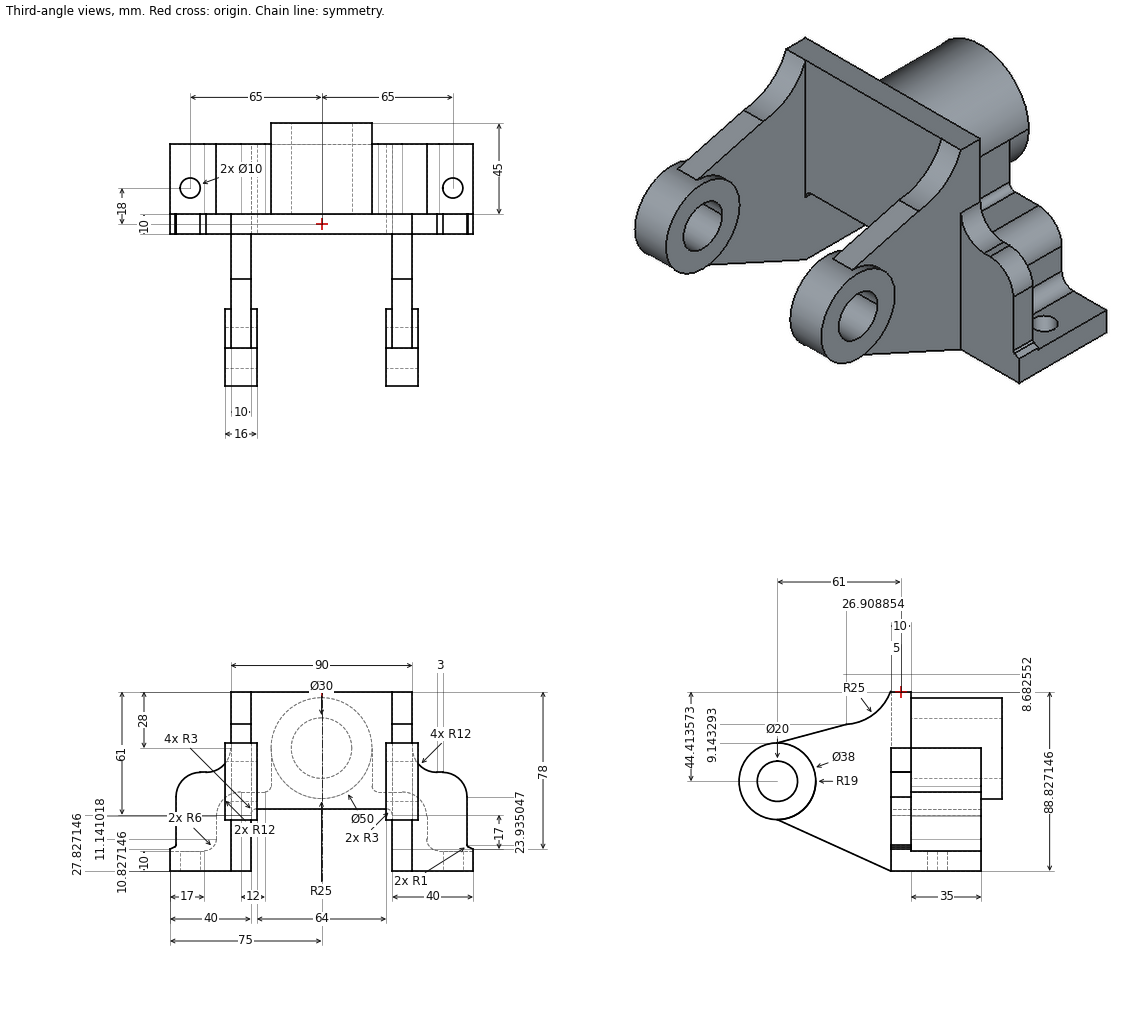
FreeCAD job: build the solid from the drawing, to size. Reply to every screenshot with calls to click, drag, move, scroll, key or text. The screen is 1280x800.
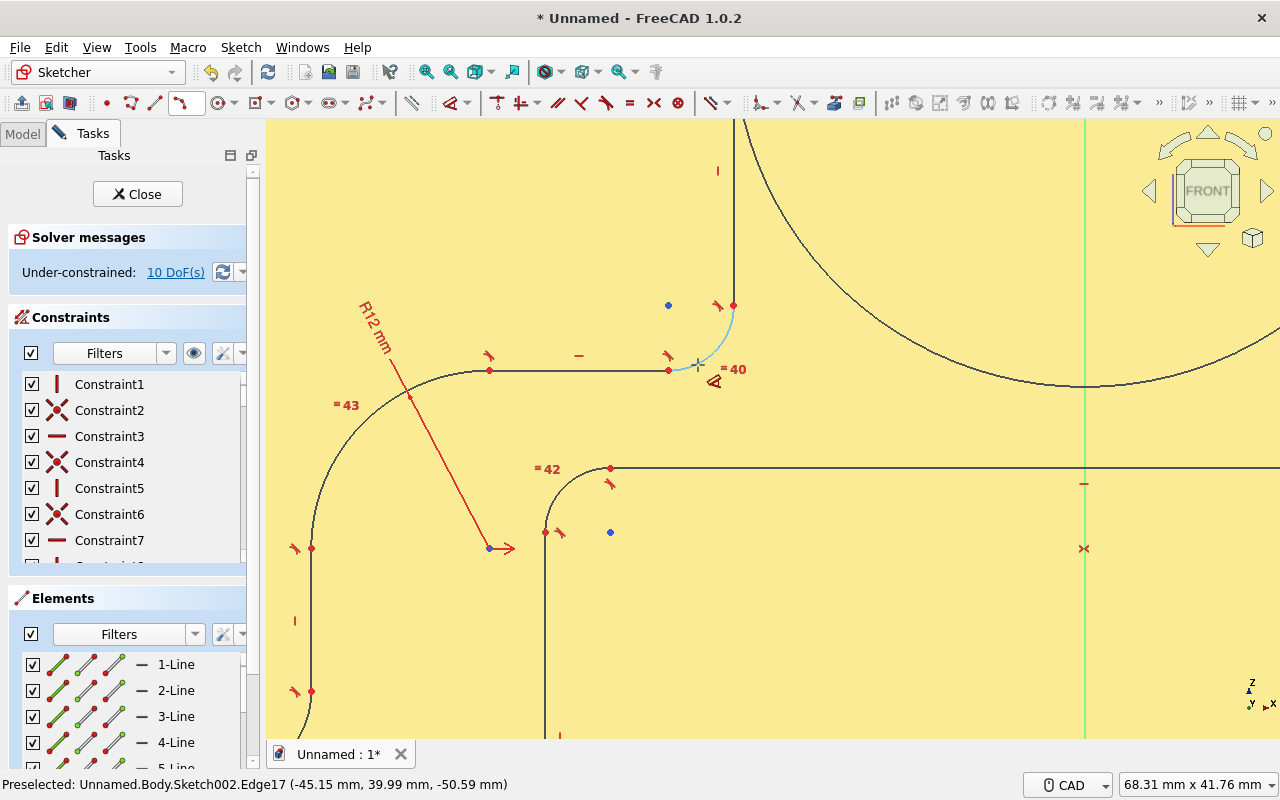
click(698, 364)
click(712, 393)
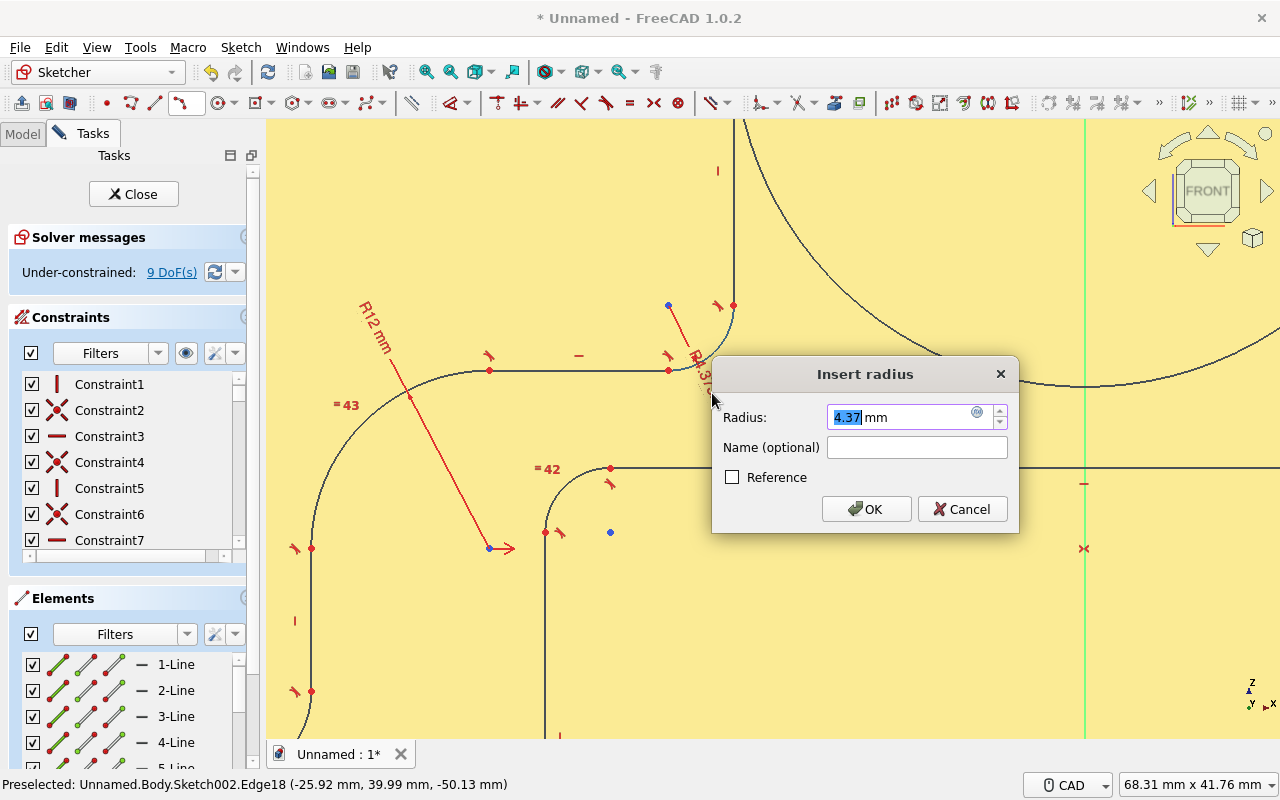
text(3)
key(Return)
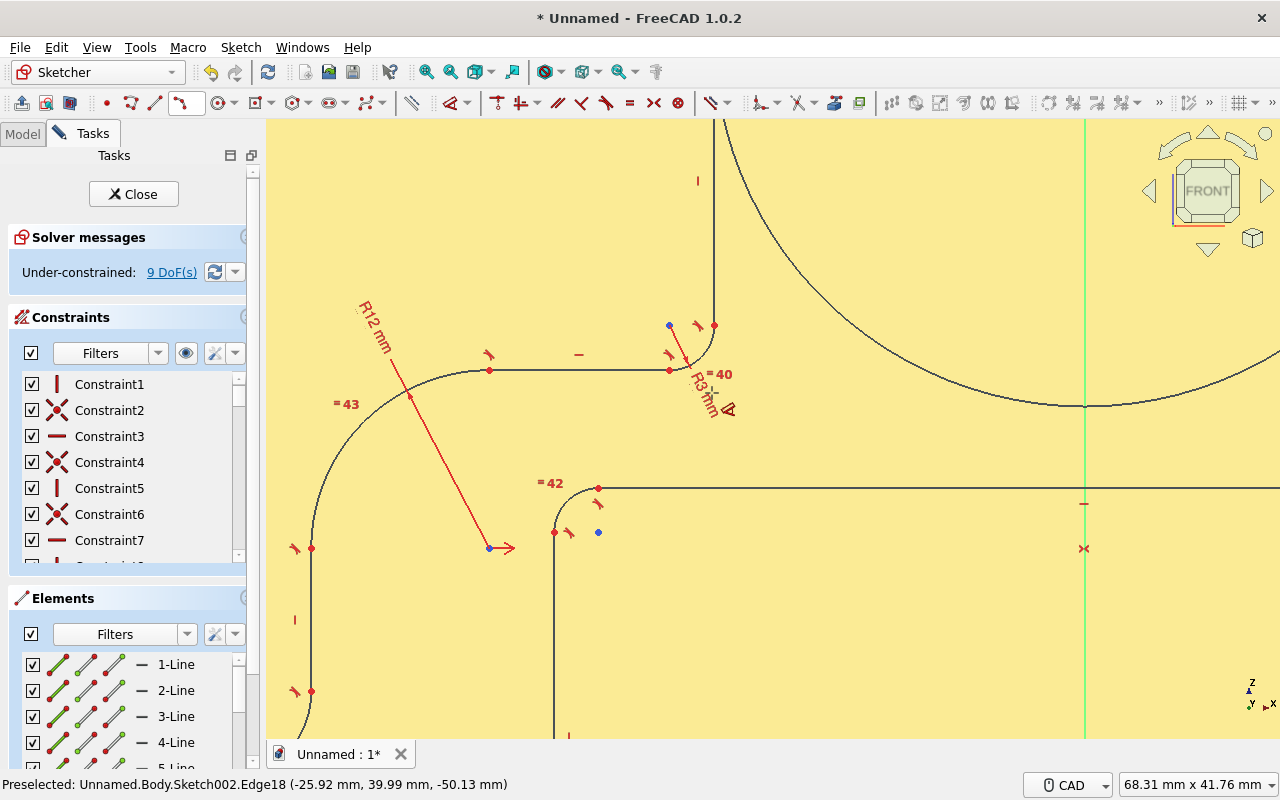
scroll(580, 479, down, 7)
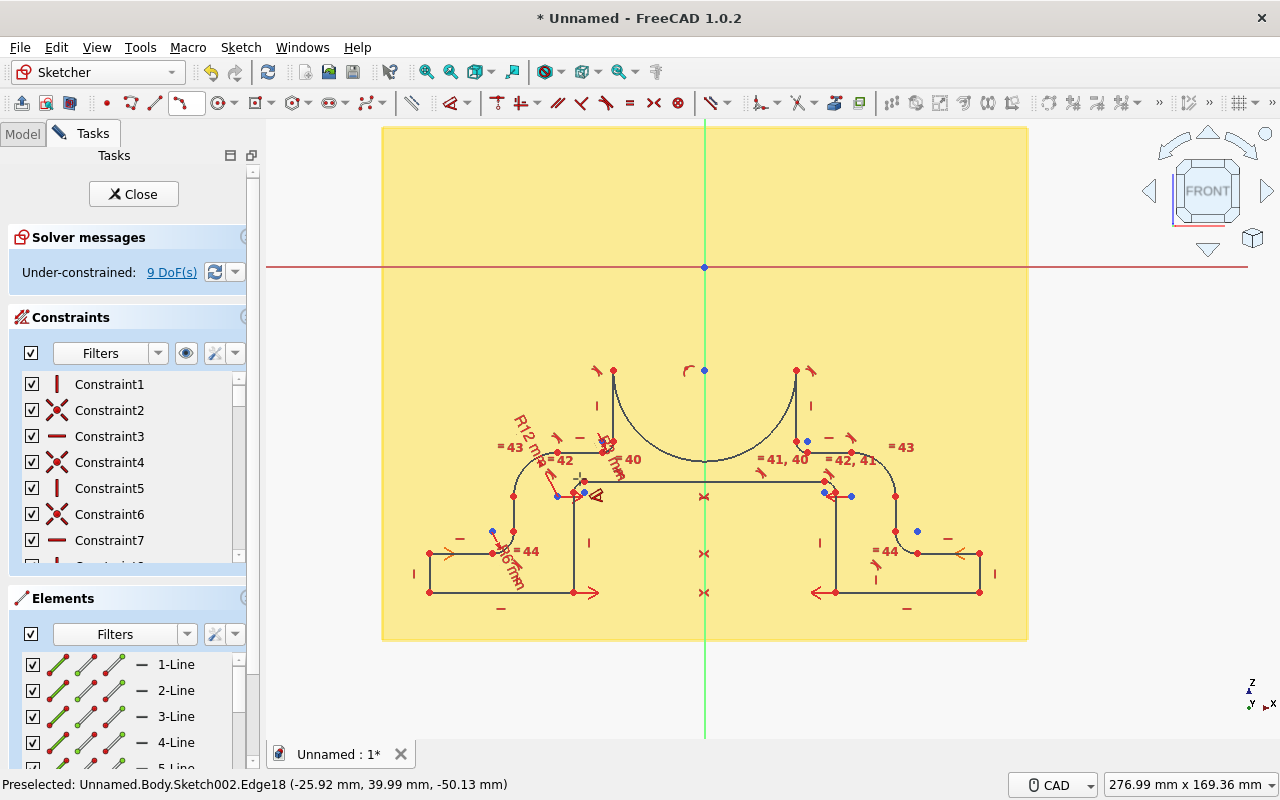
click(651, 444)
click(582, 363)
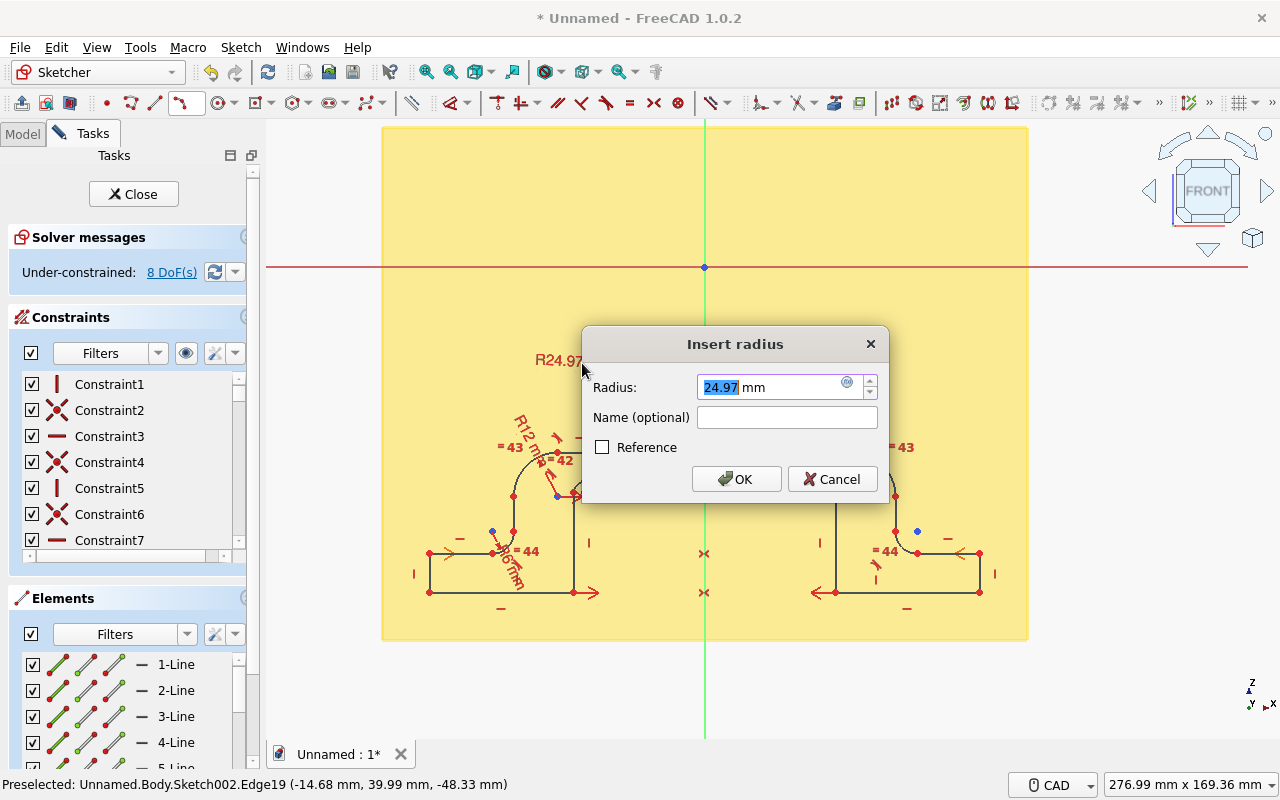
text(25)
key(Return)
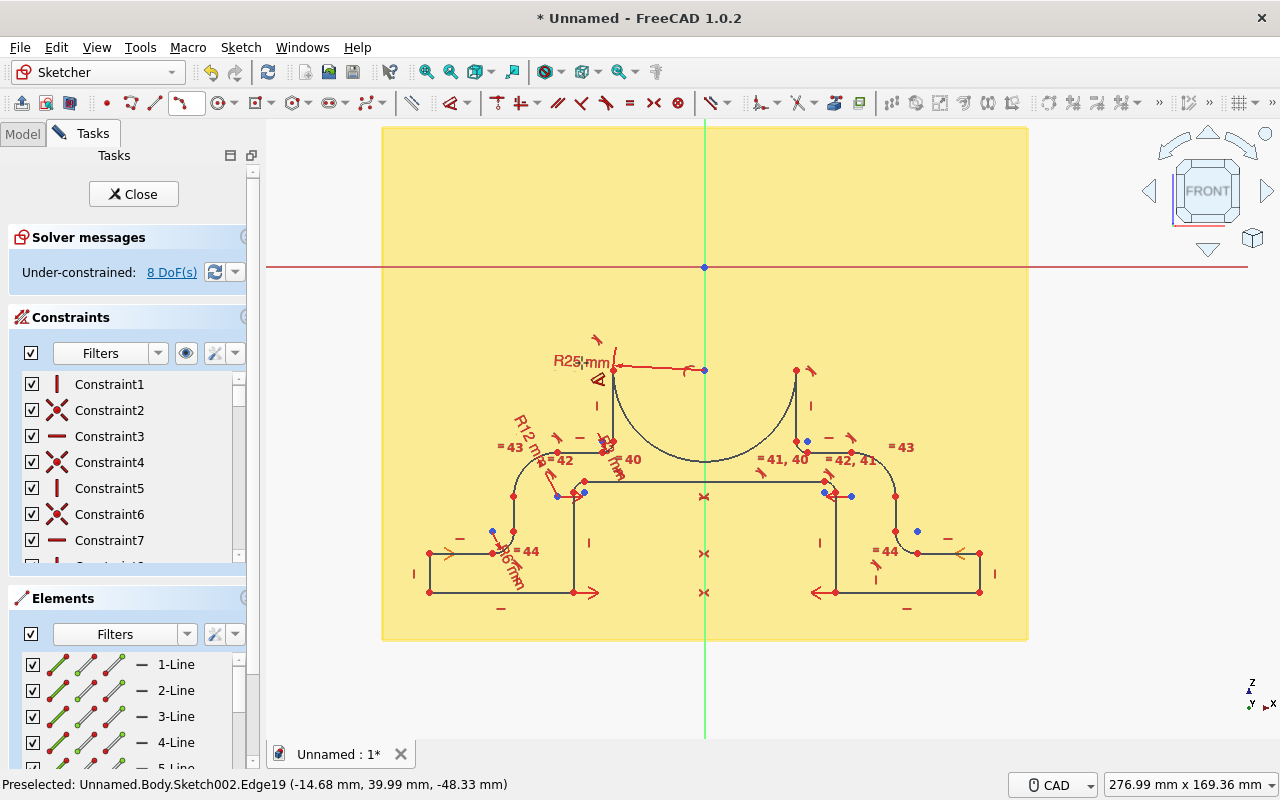
click(531, 593)
click(502, 627)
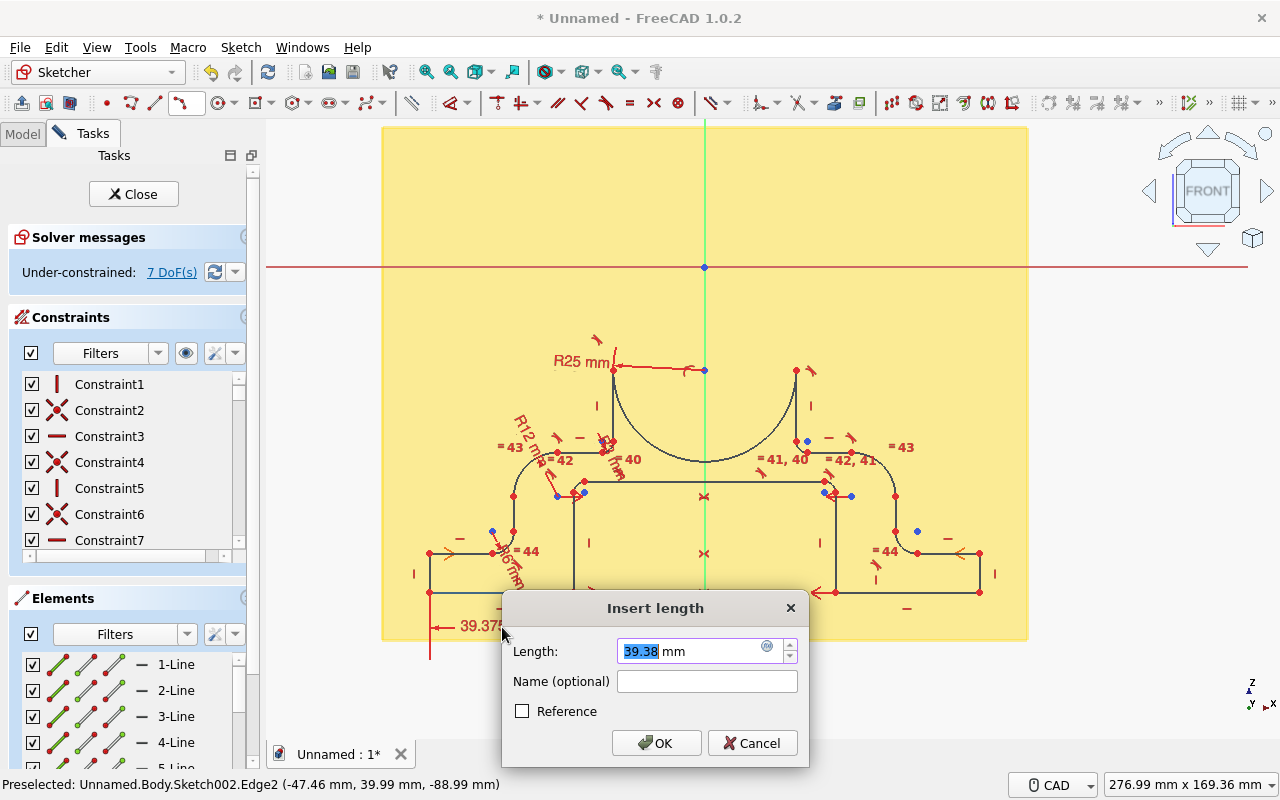
text(40)
key(Return)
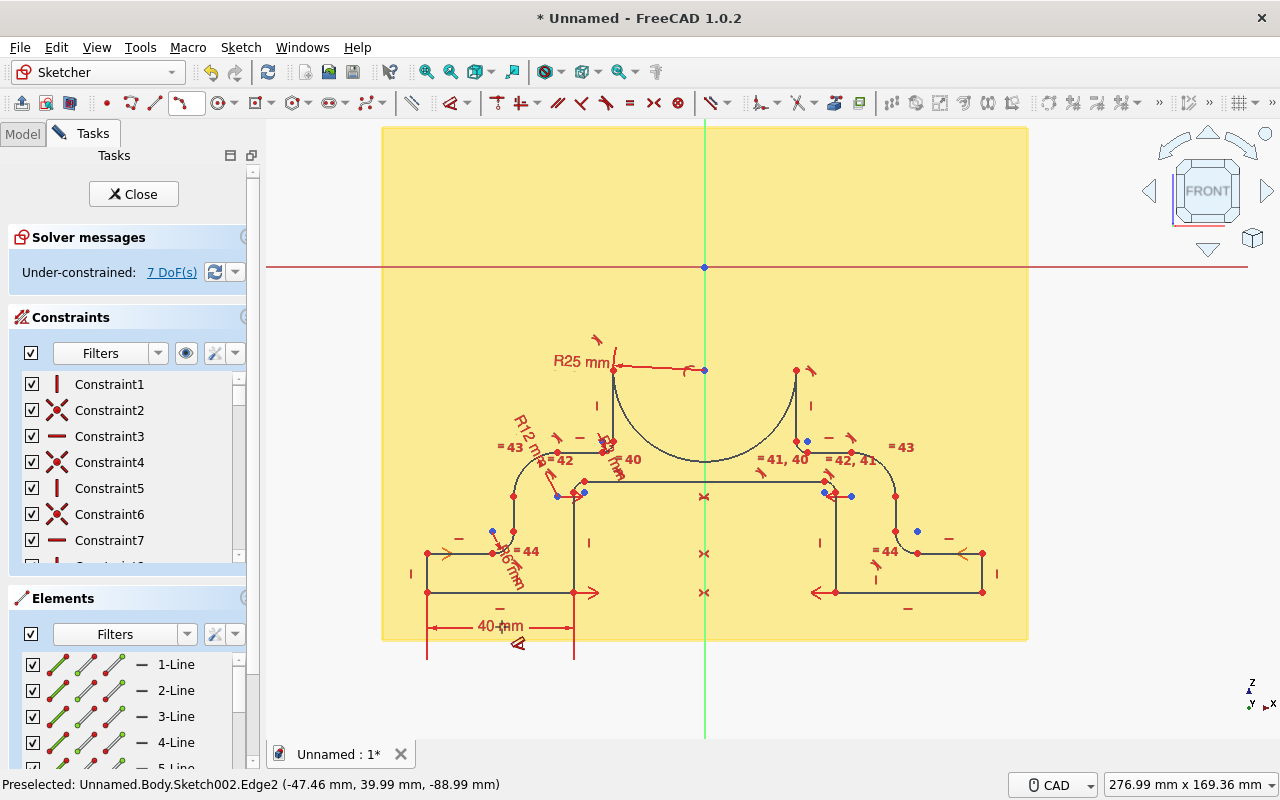
click(427, 581)
click(393, 573)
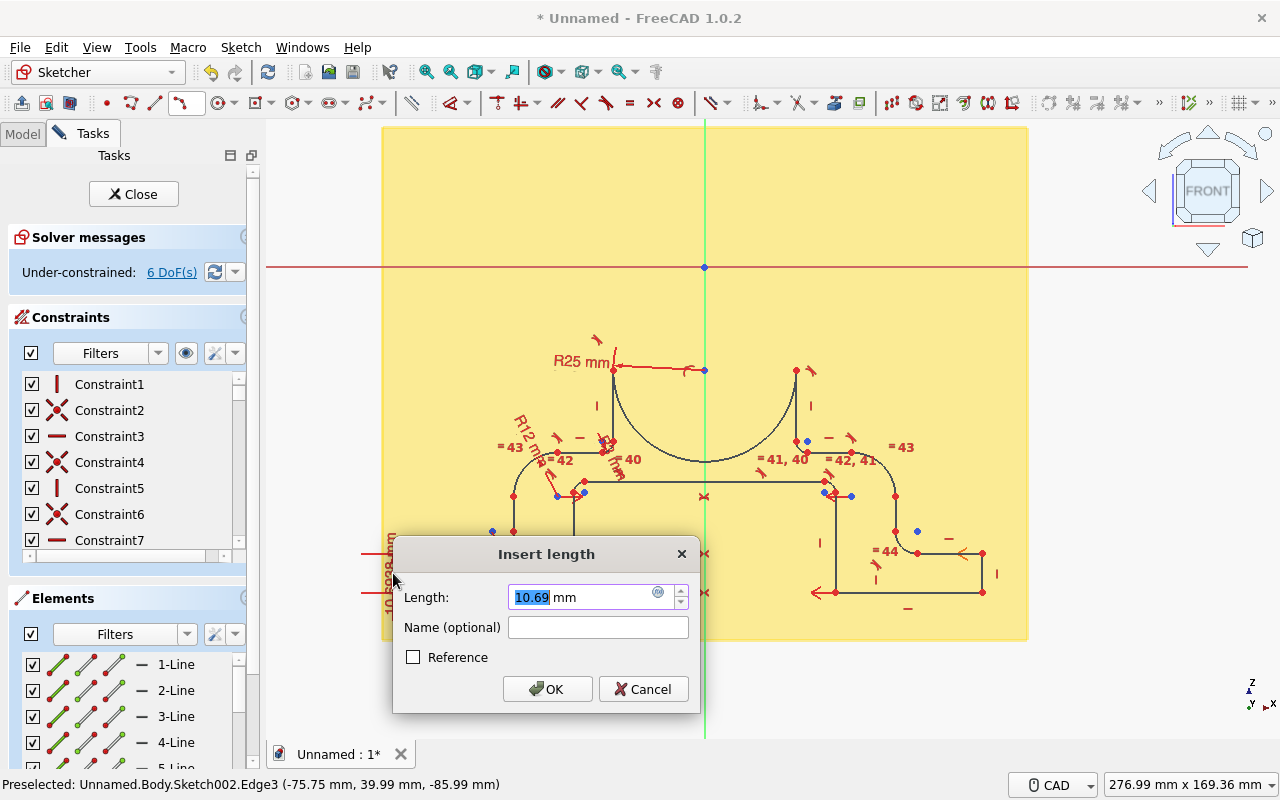
text(10)
key(Return)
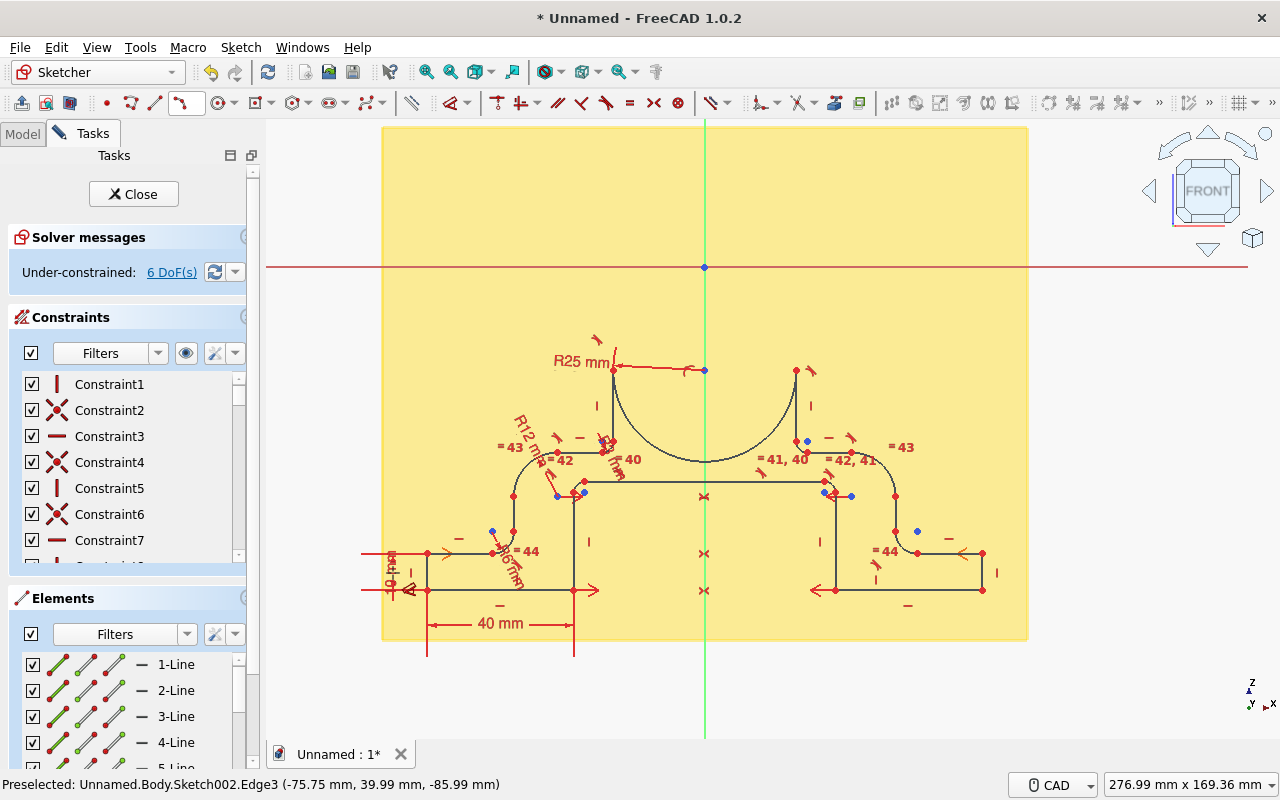
click(447, 554)
click(460, 520)